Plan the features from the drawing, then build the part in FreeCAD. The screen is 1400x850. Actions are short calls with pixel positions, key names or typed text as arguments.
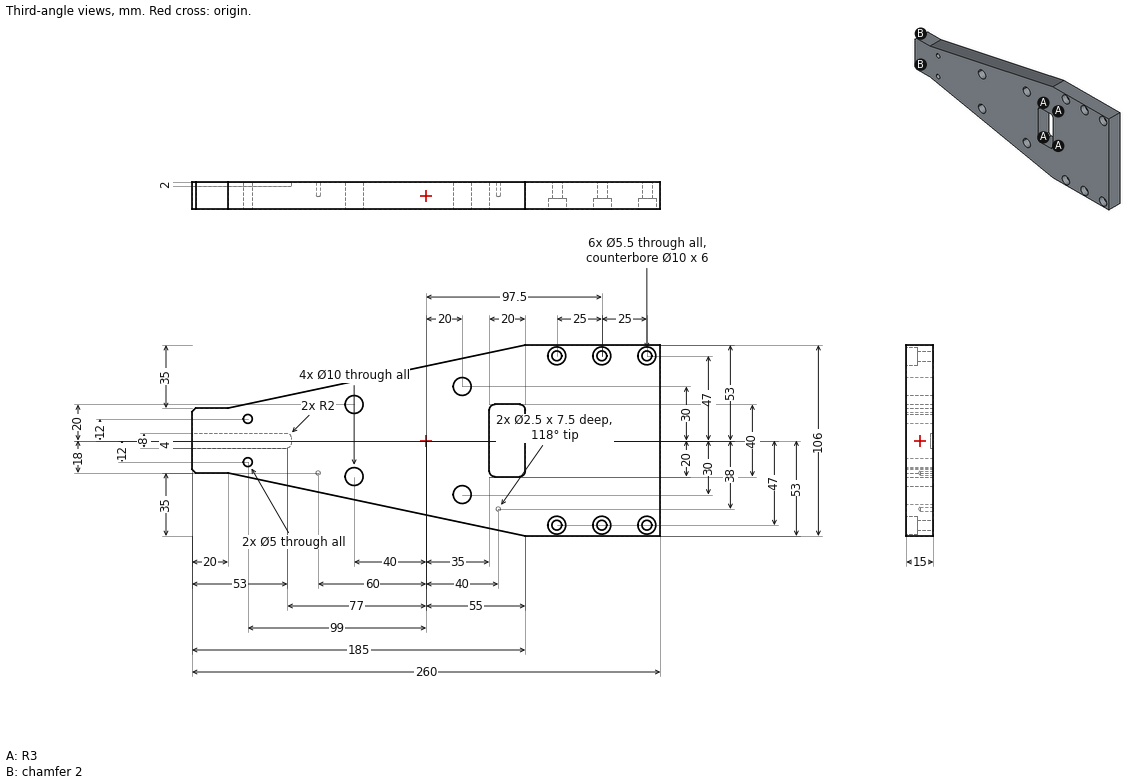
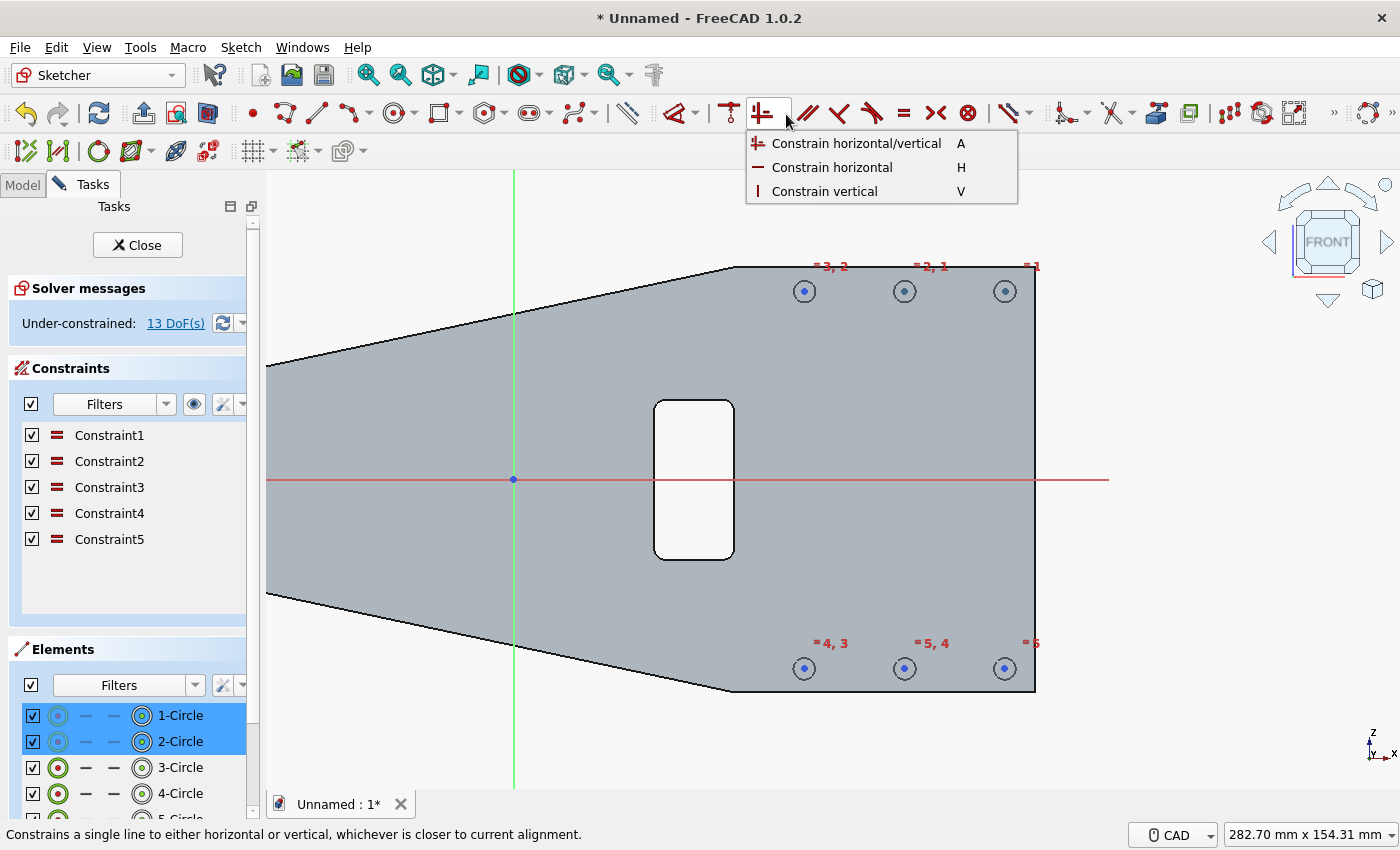
click(882, 167)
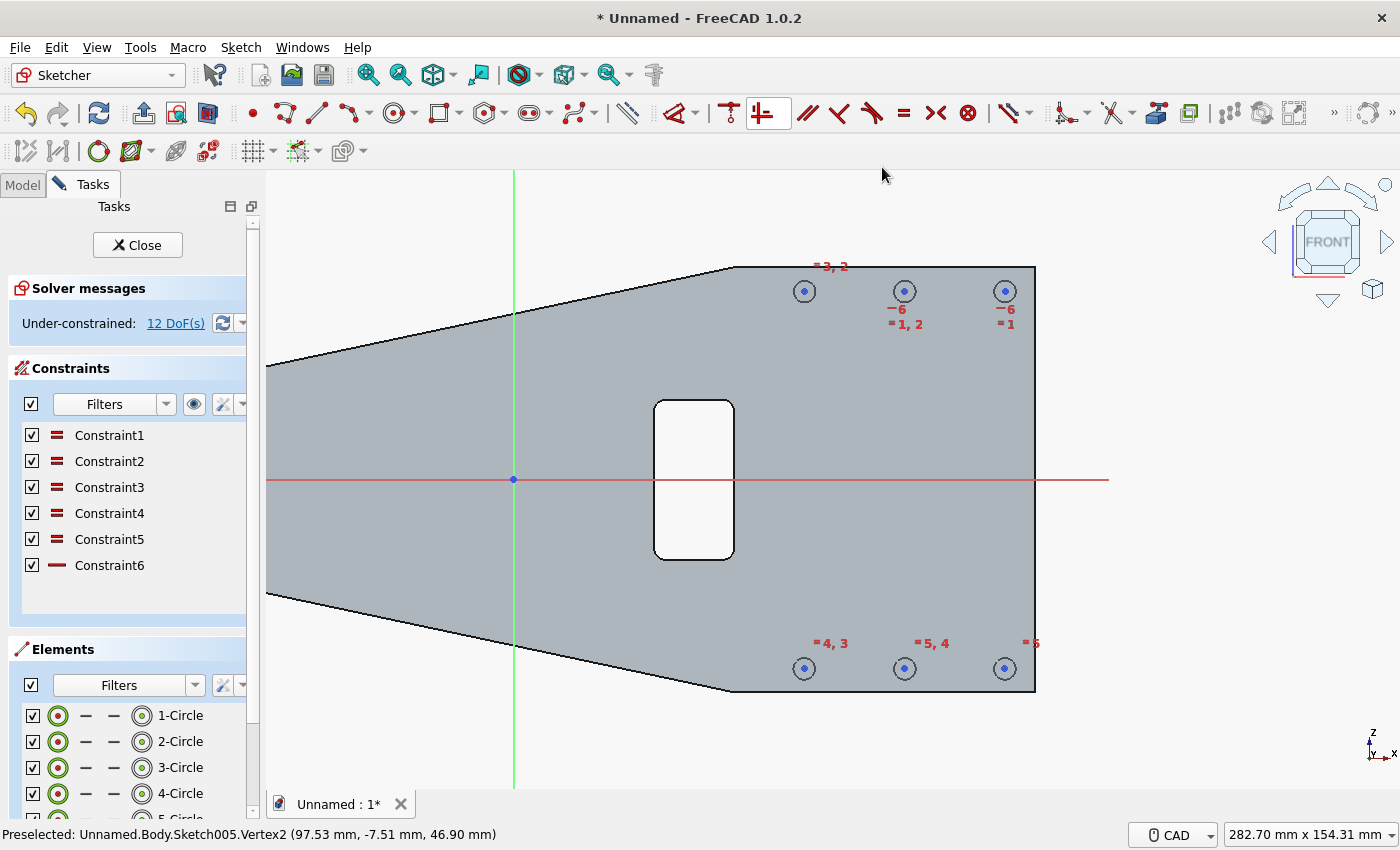
click(905, 292)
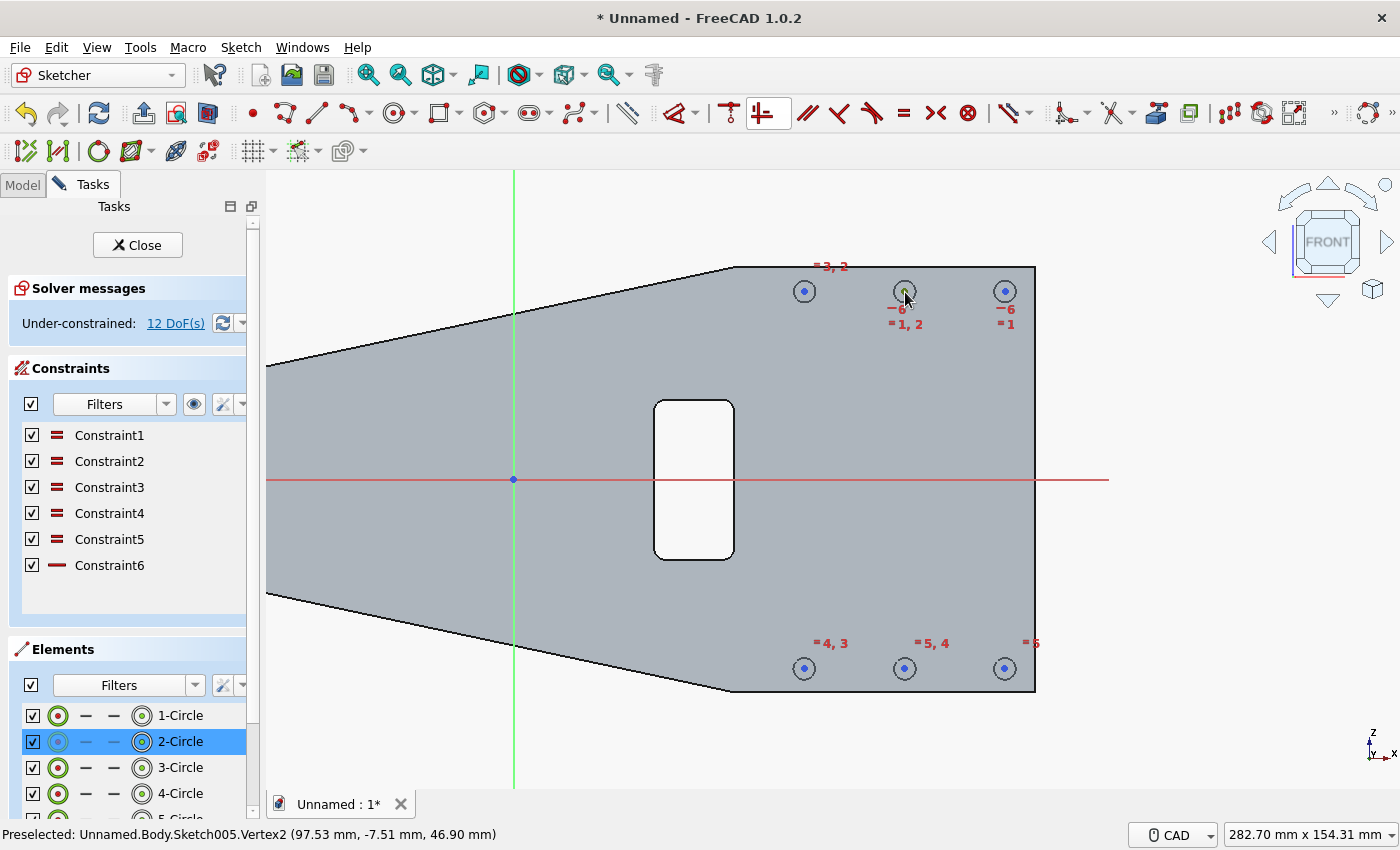
click(805, 292)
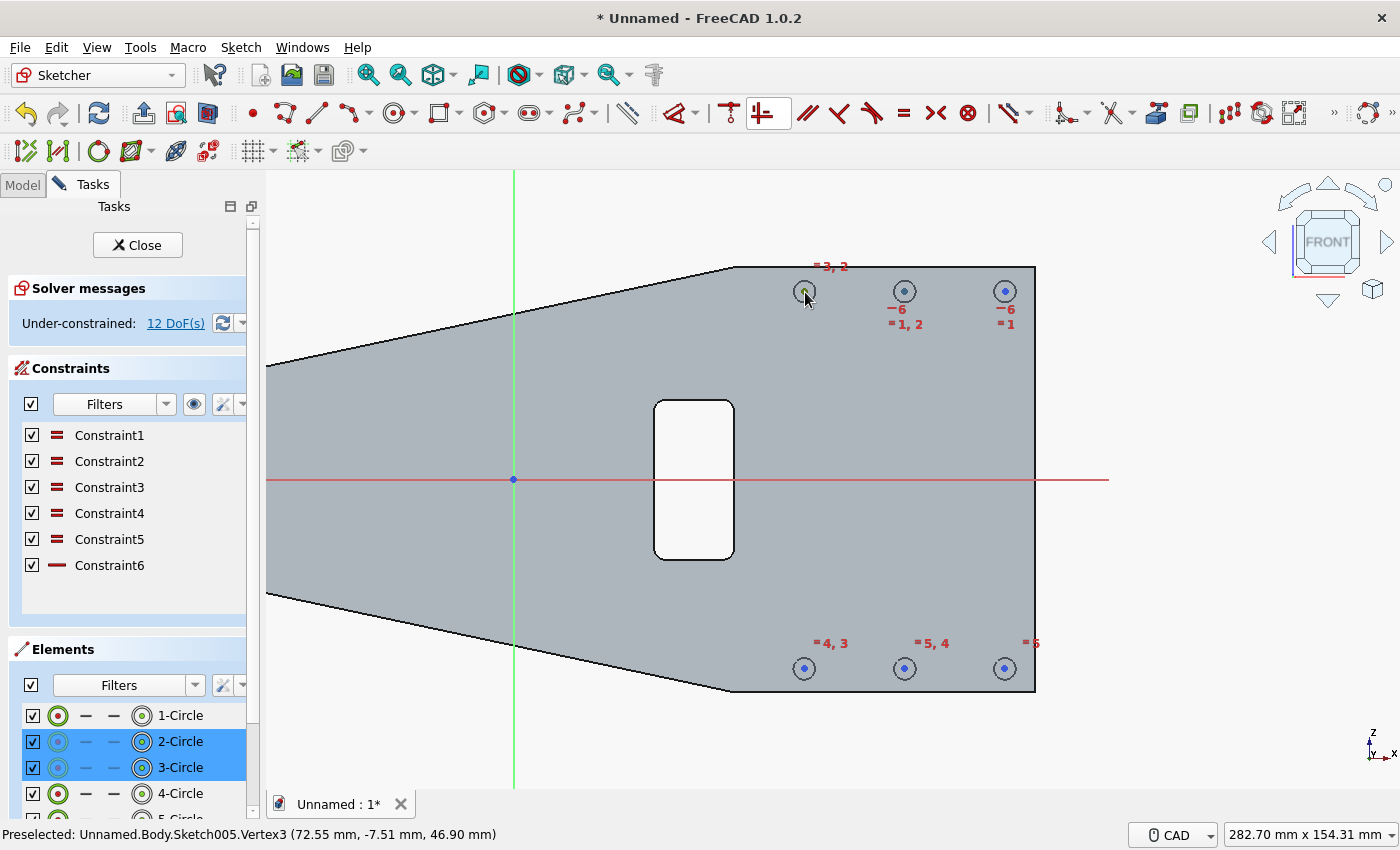
key(h)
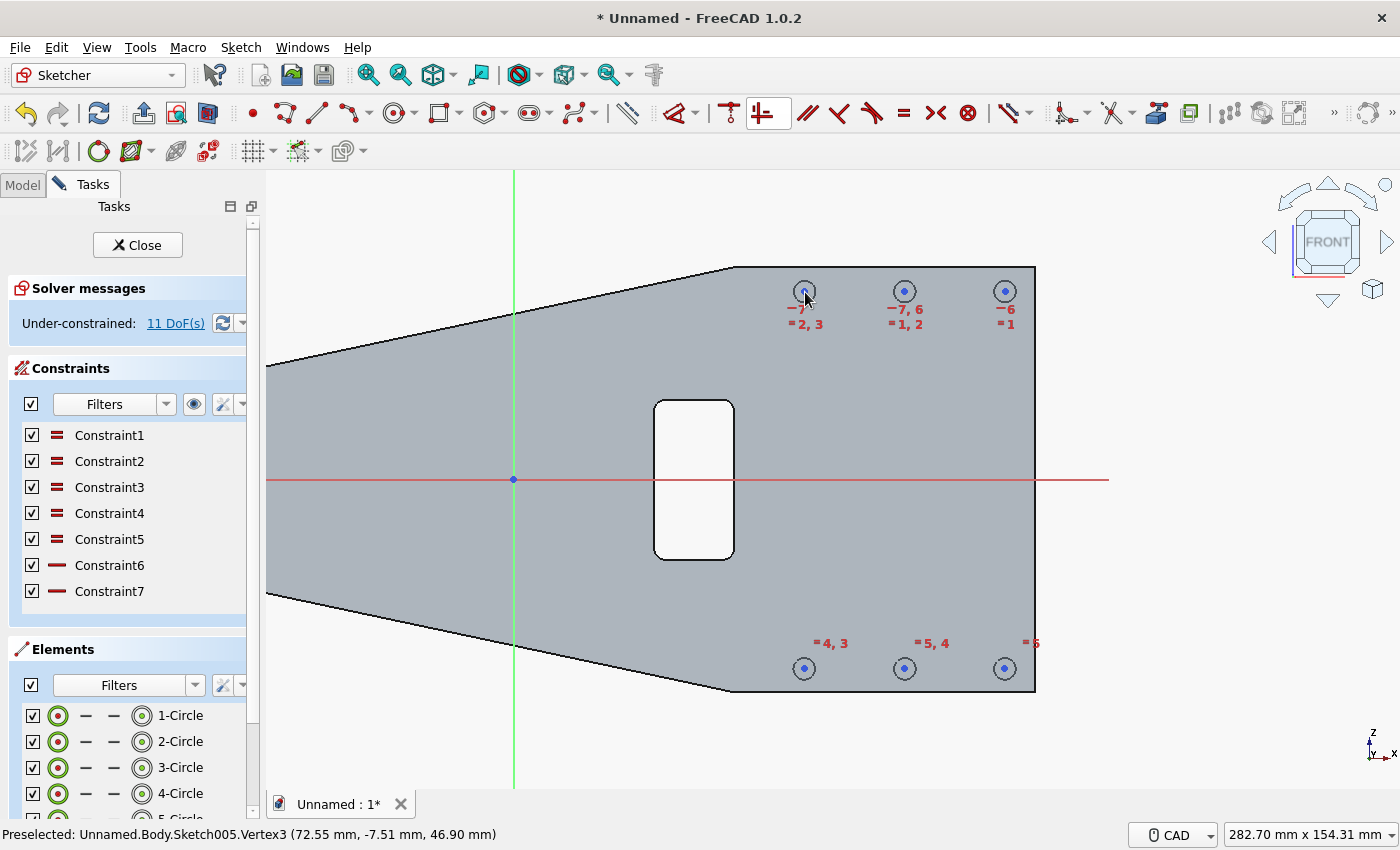
click(805, 292)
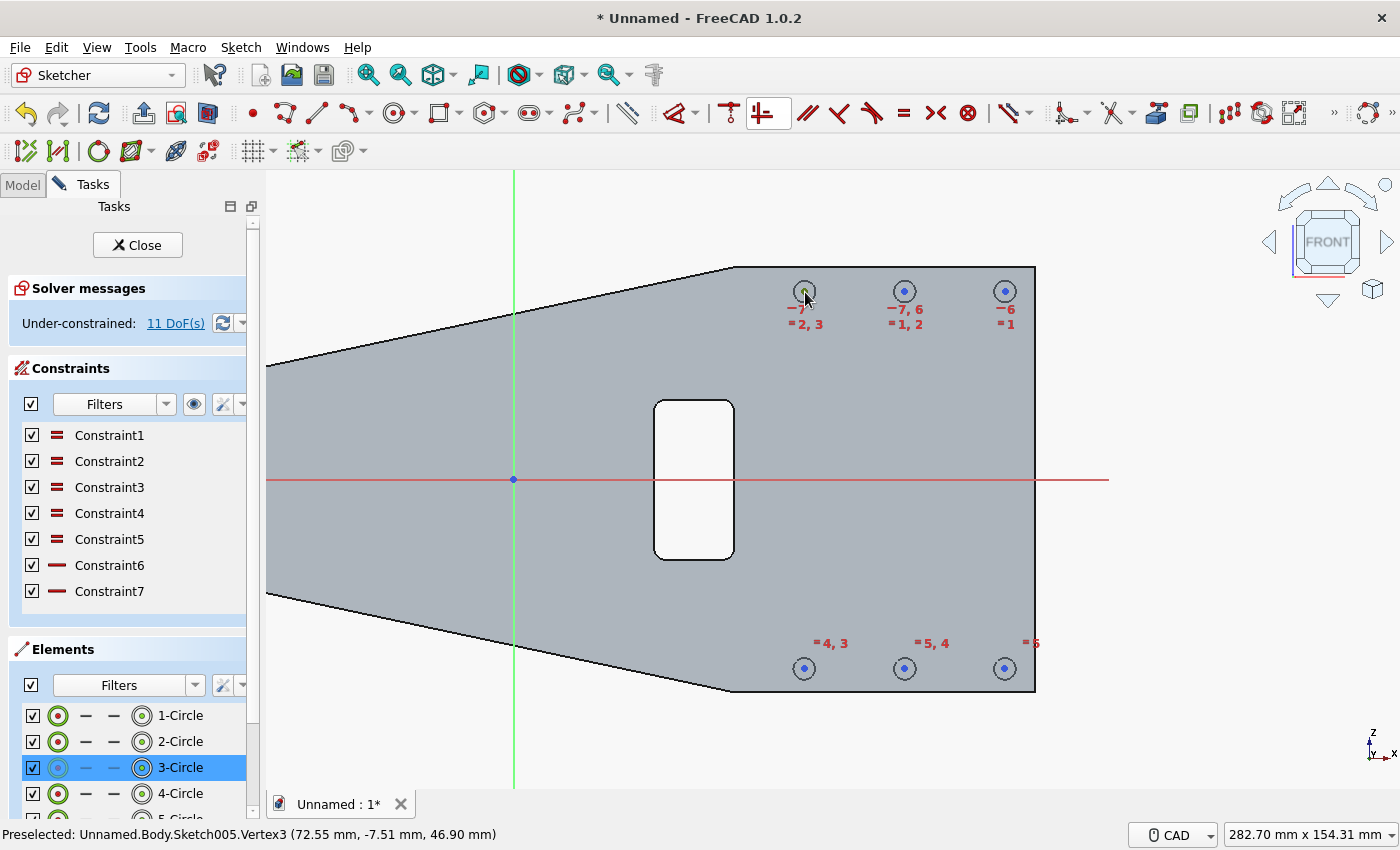
click(804, 669)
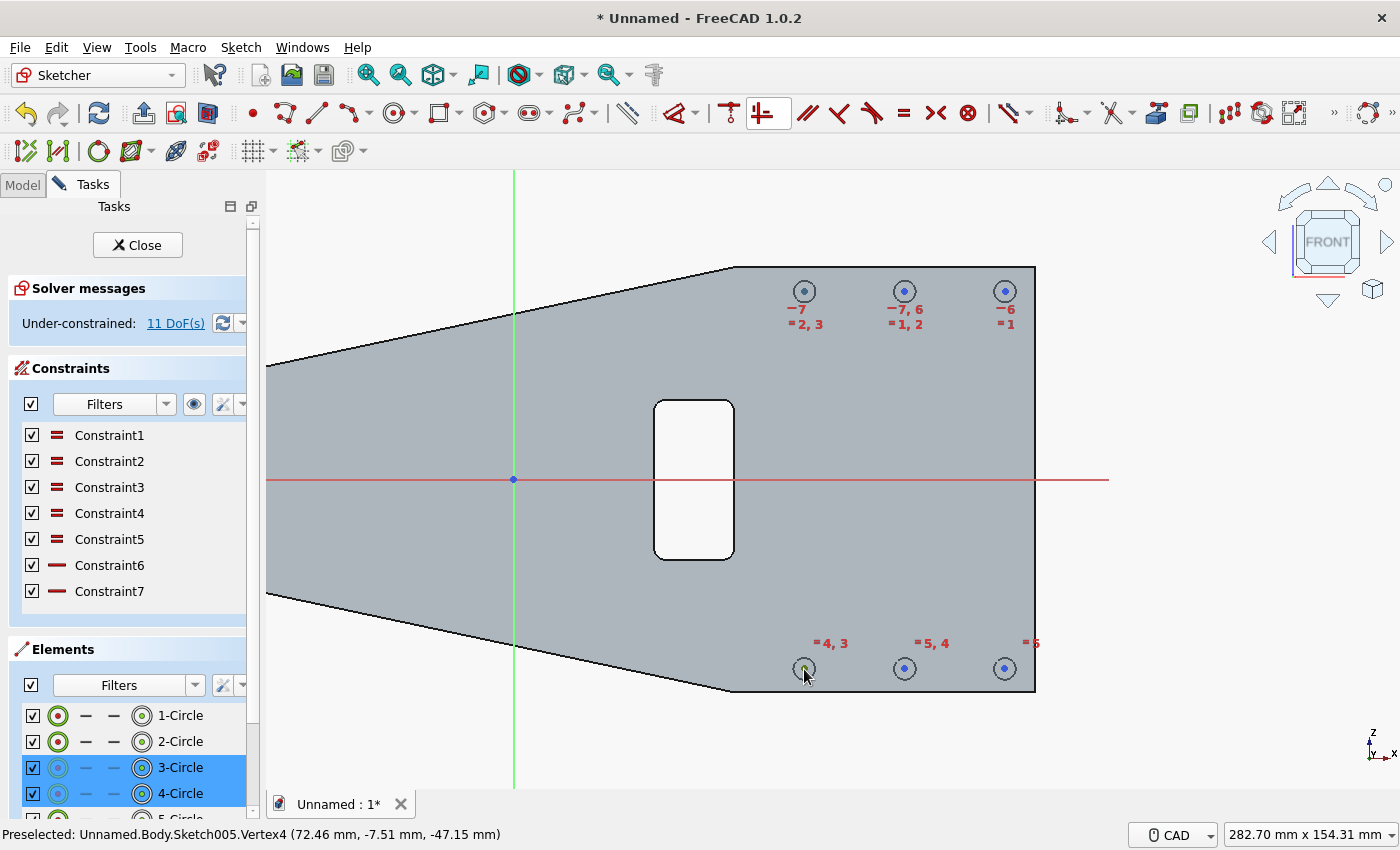
key(v)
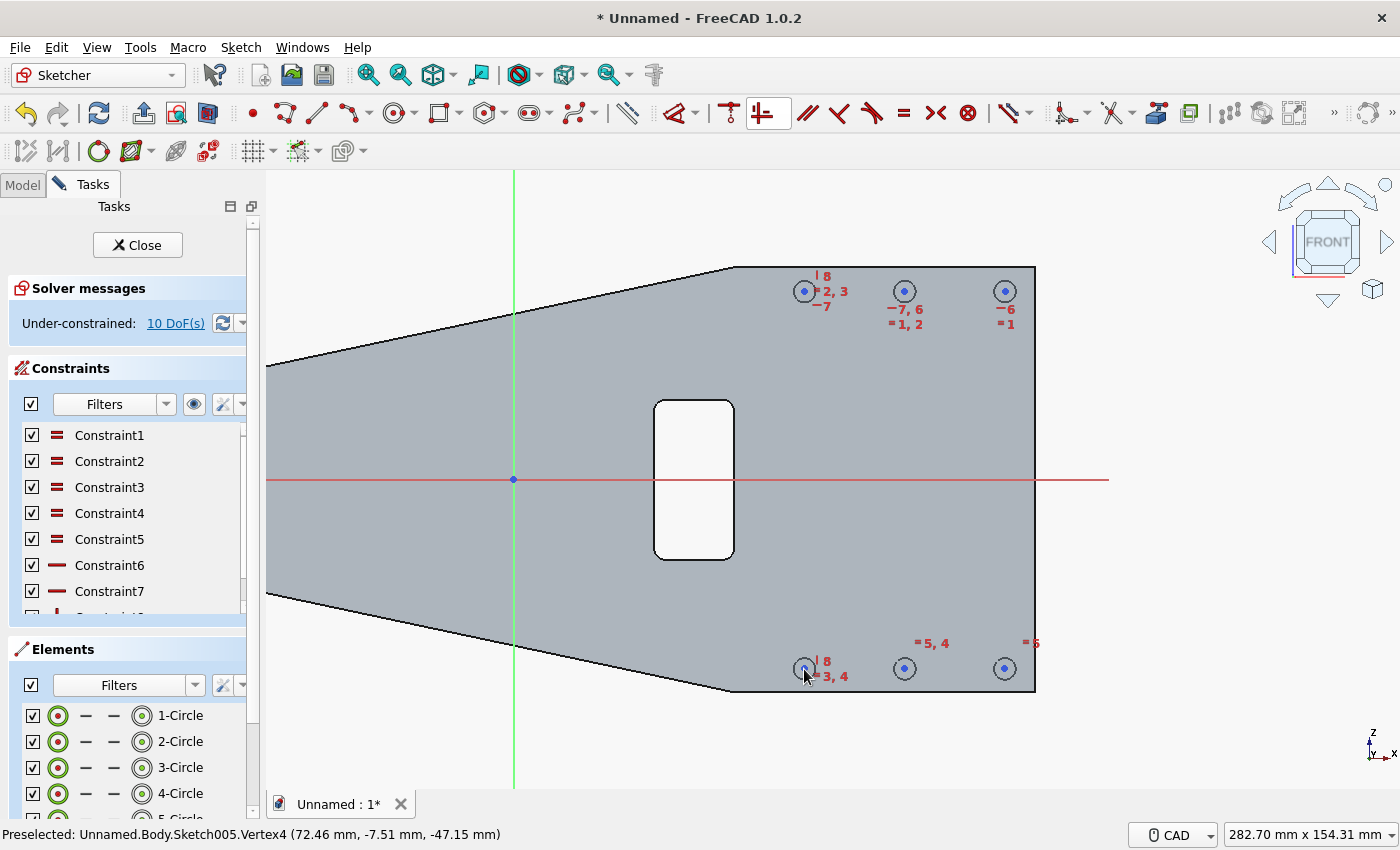
click(905, 292)